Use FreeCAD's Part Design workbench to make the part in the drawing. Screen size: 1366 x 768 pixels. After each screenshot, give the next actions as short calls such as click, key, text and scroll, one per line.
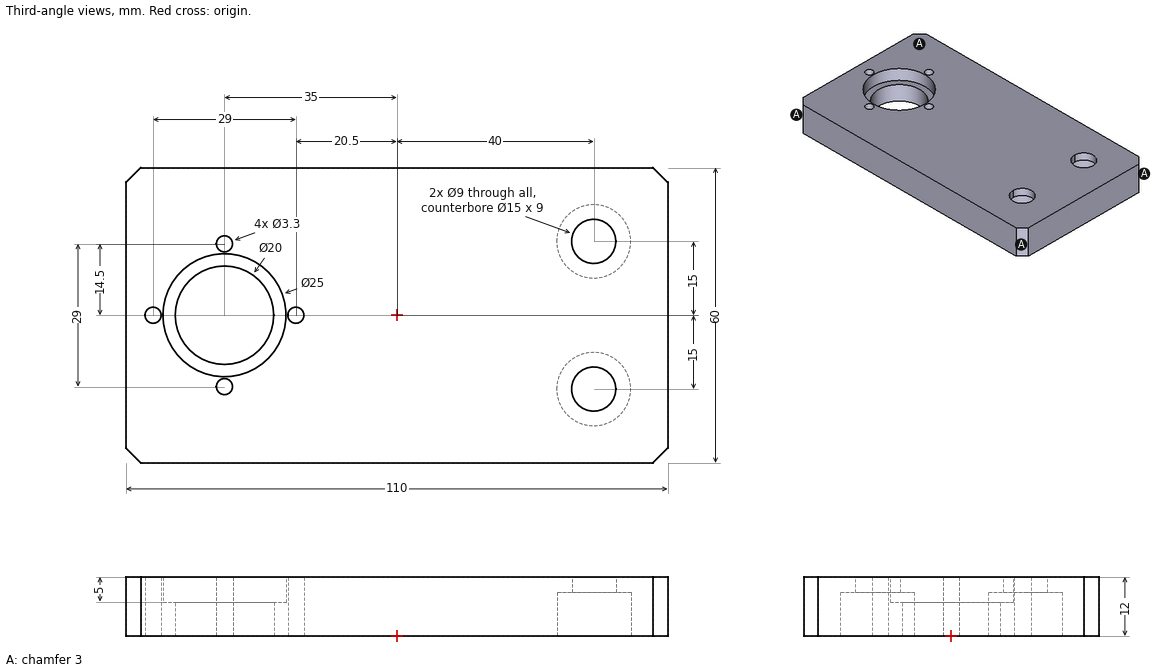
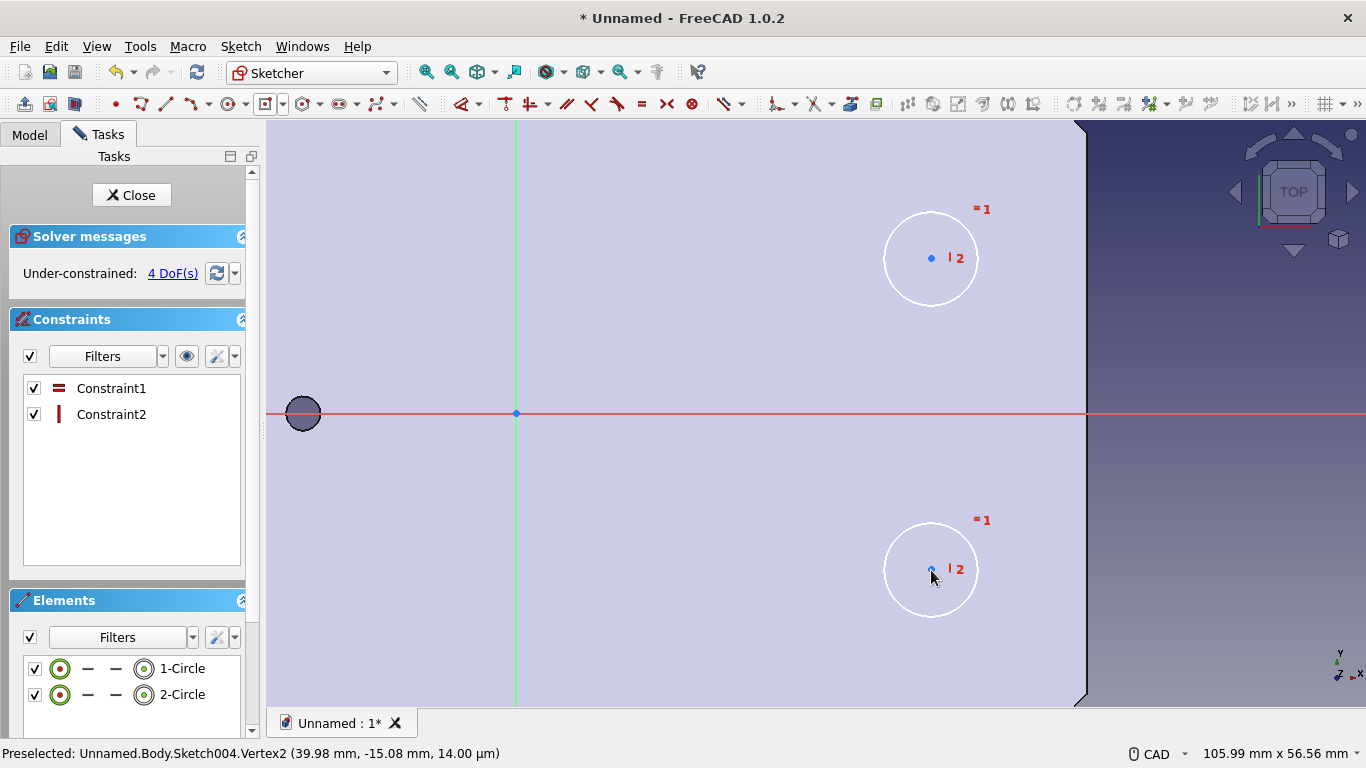
click(460, 104)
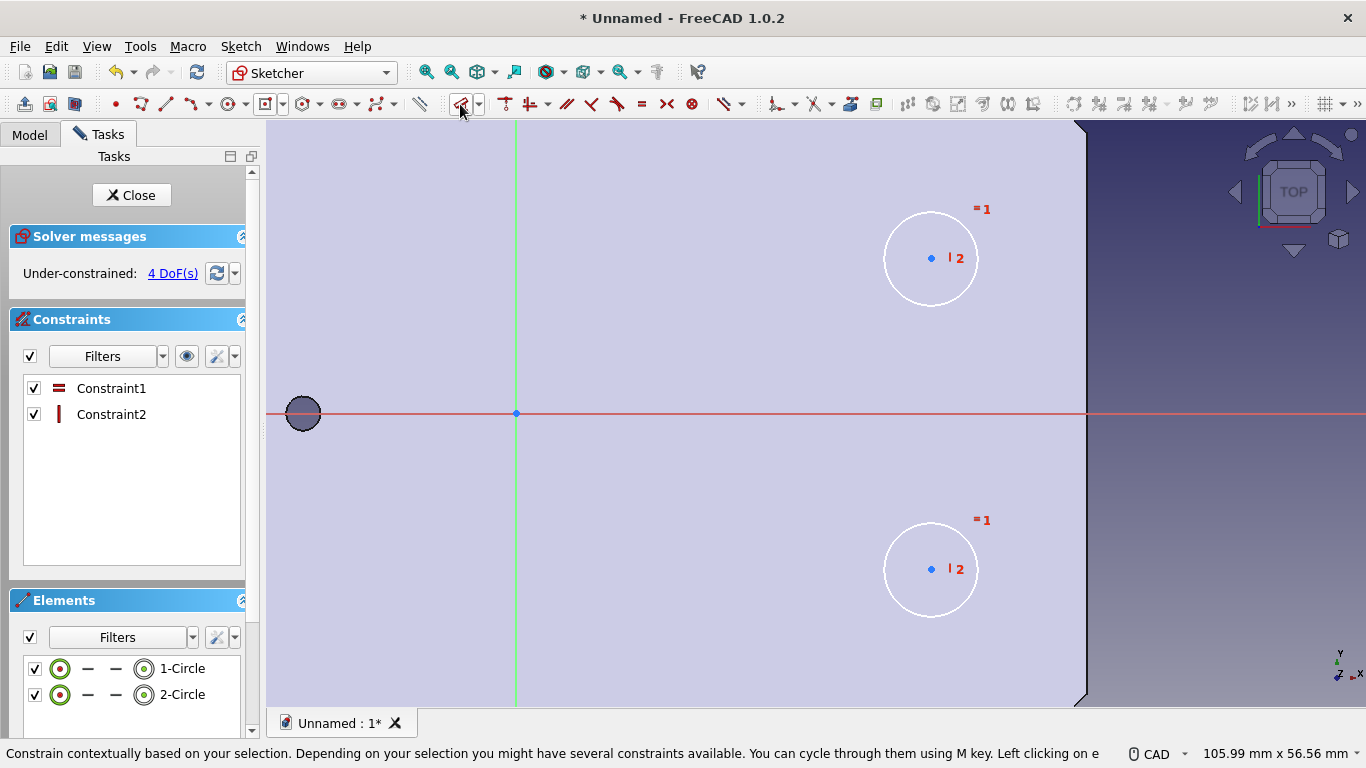
click(964, 226)
click(987, 203)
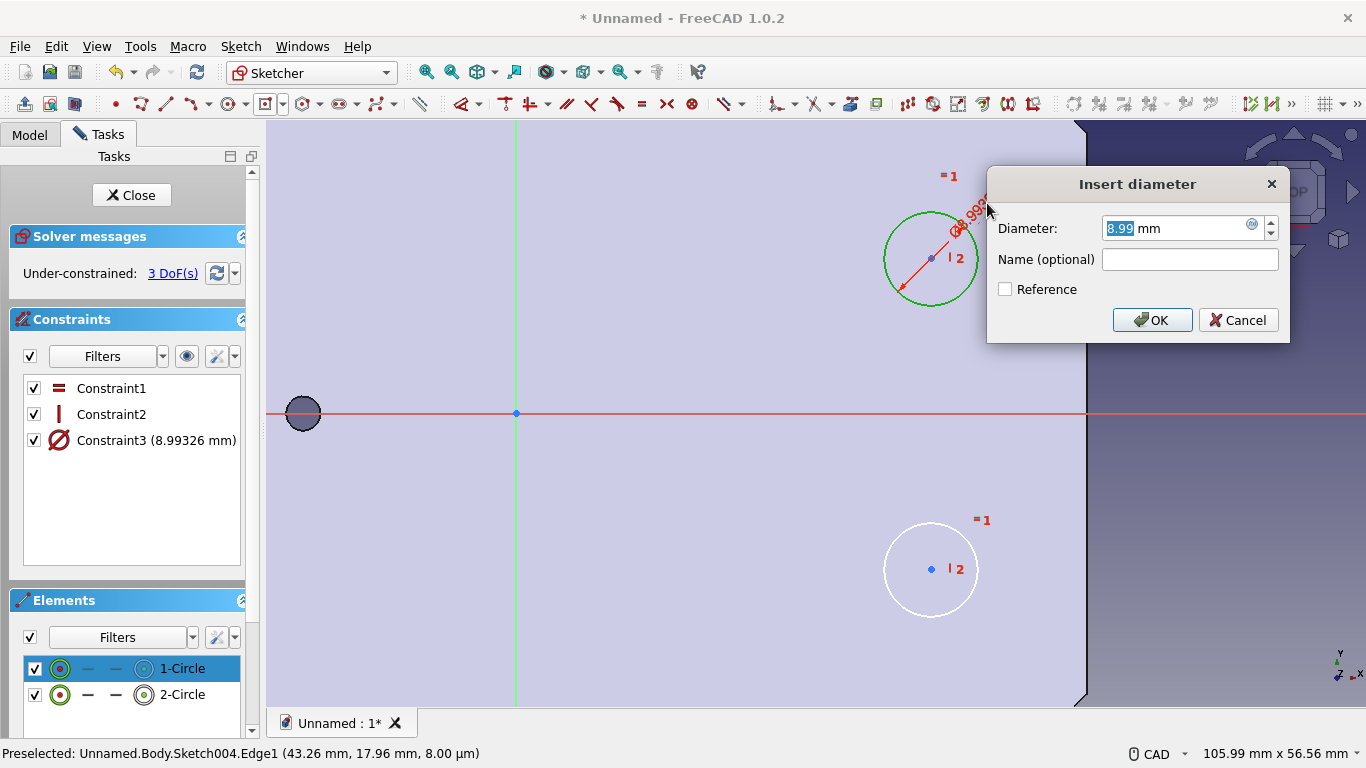
text(9)
key(Return)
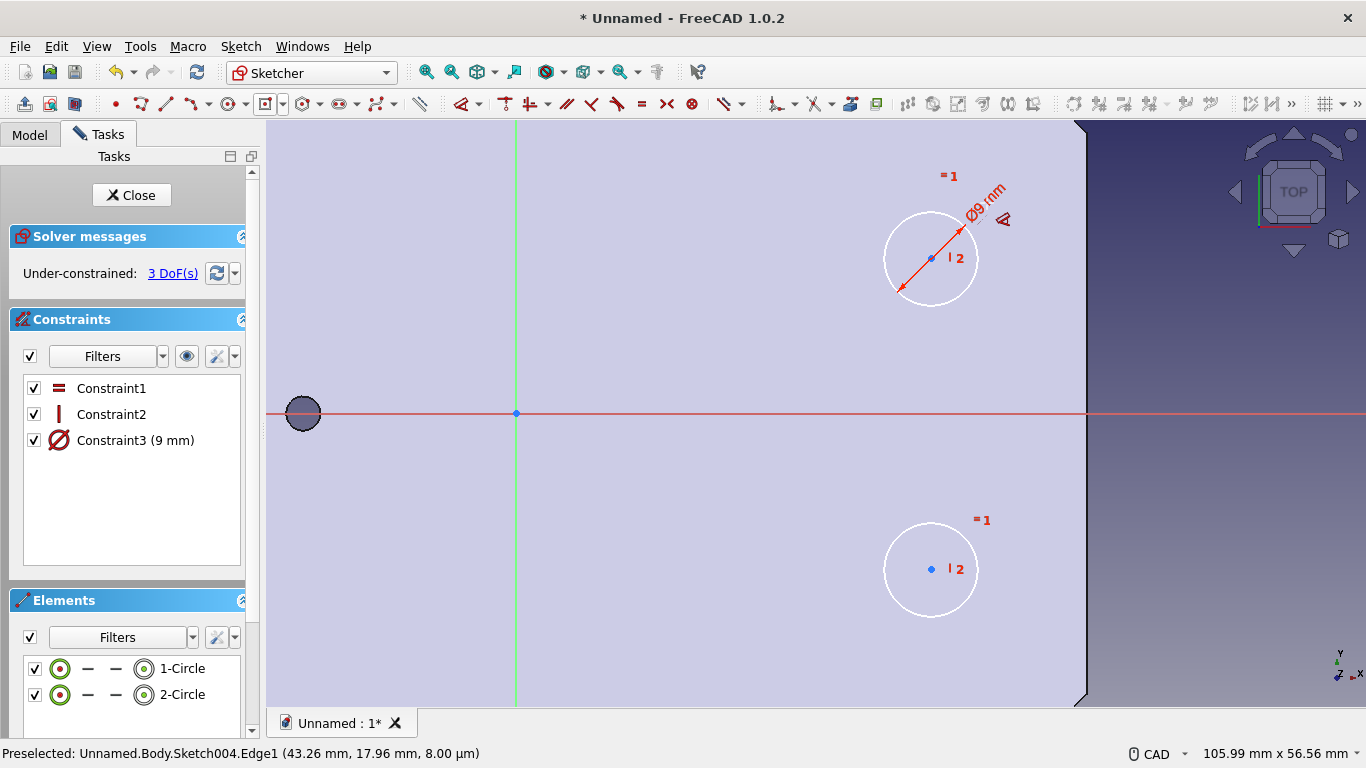
click(931, 259)
click(724, 225)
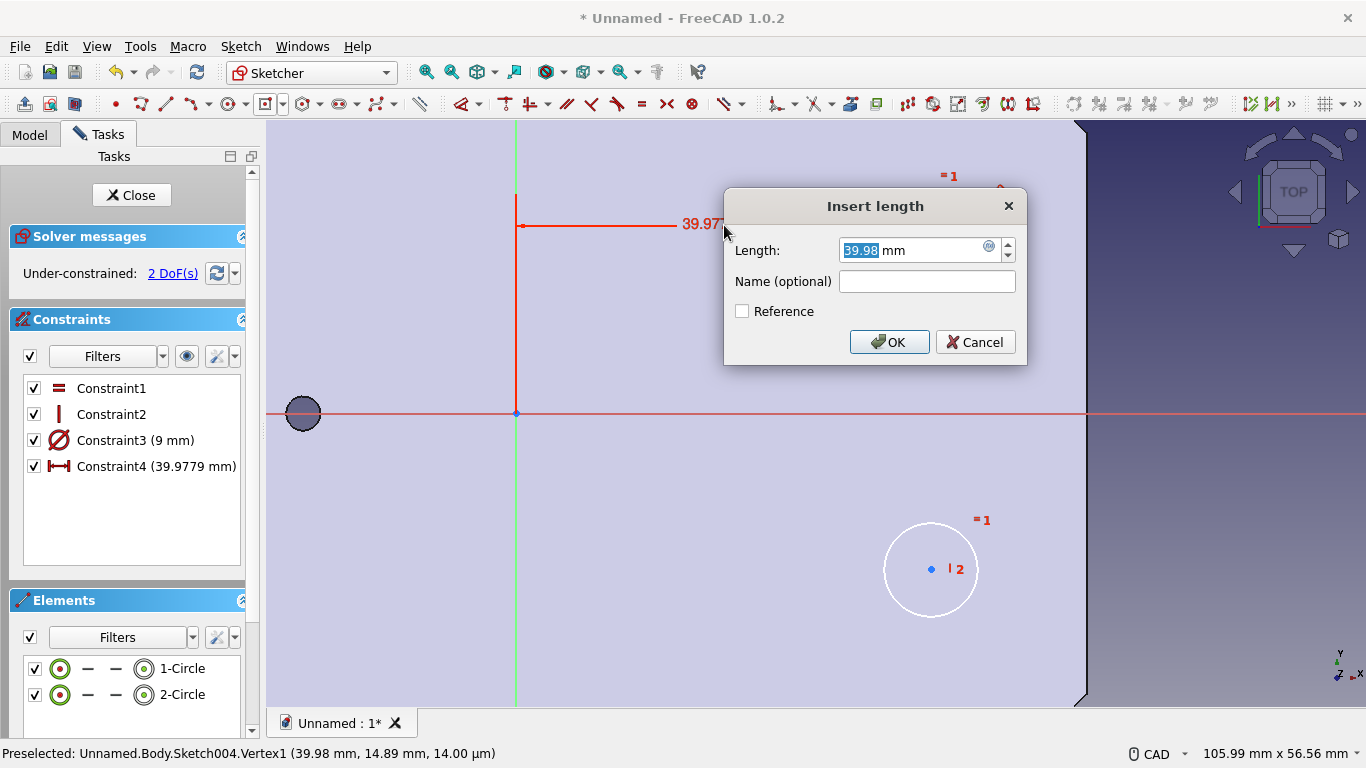
text(40)
key(Return)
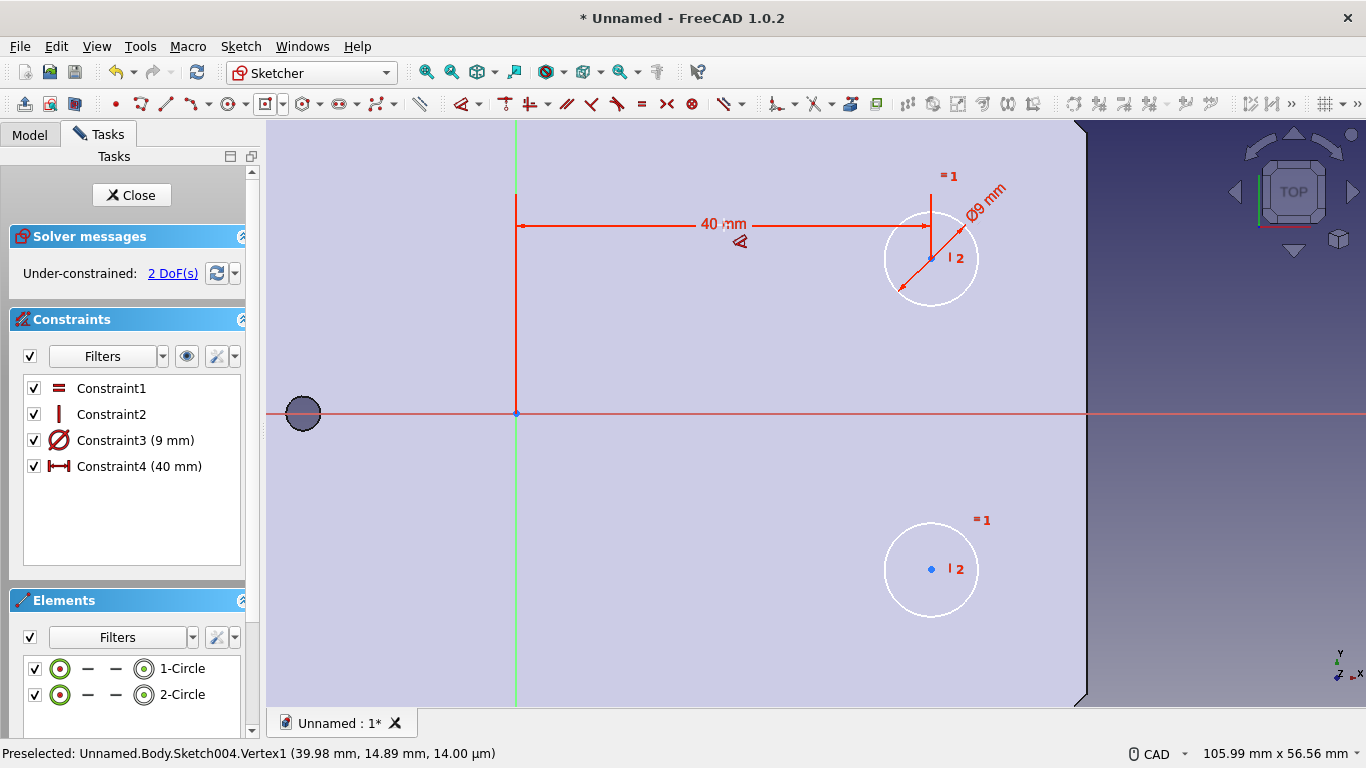
click(931, 259)
click(482, 336)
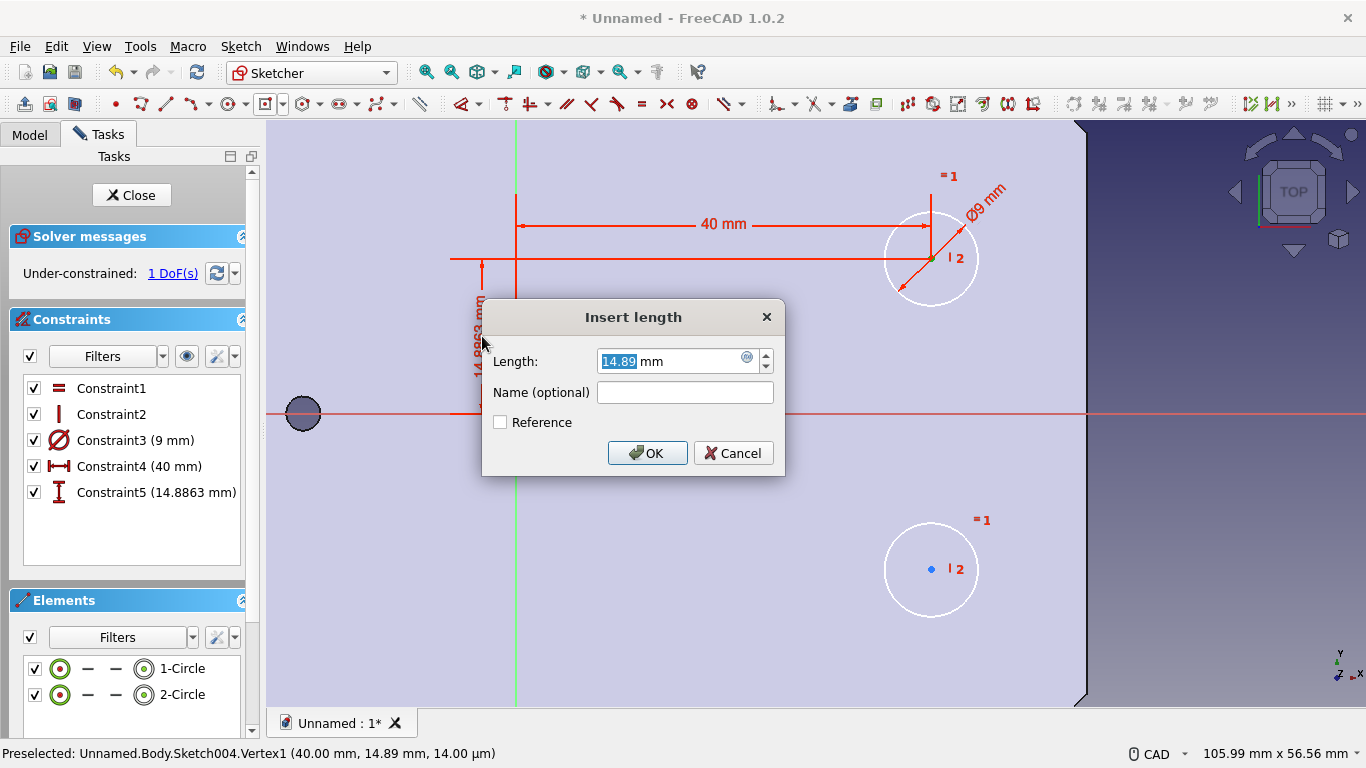
text(15)
key(Return)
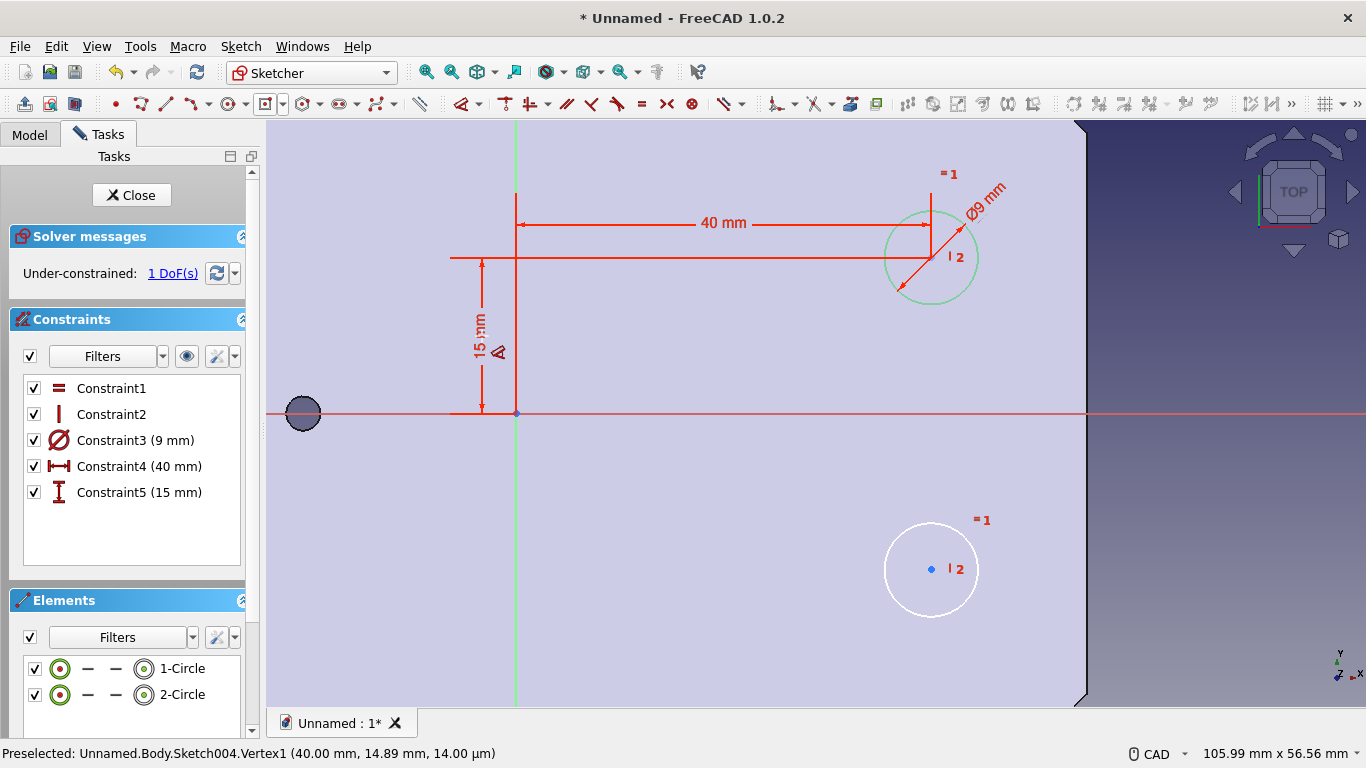
click(931, 570)
click(482, 492)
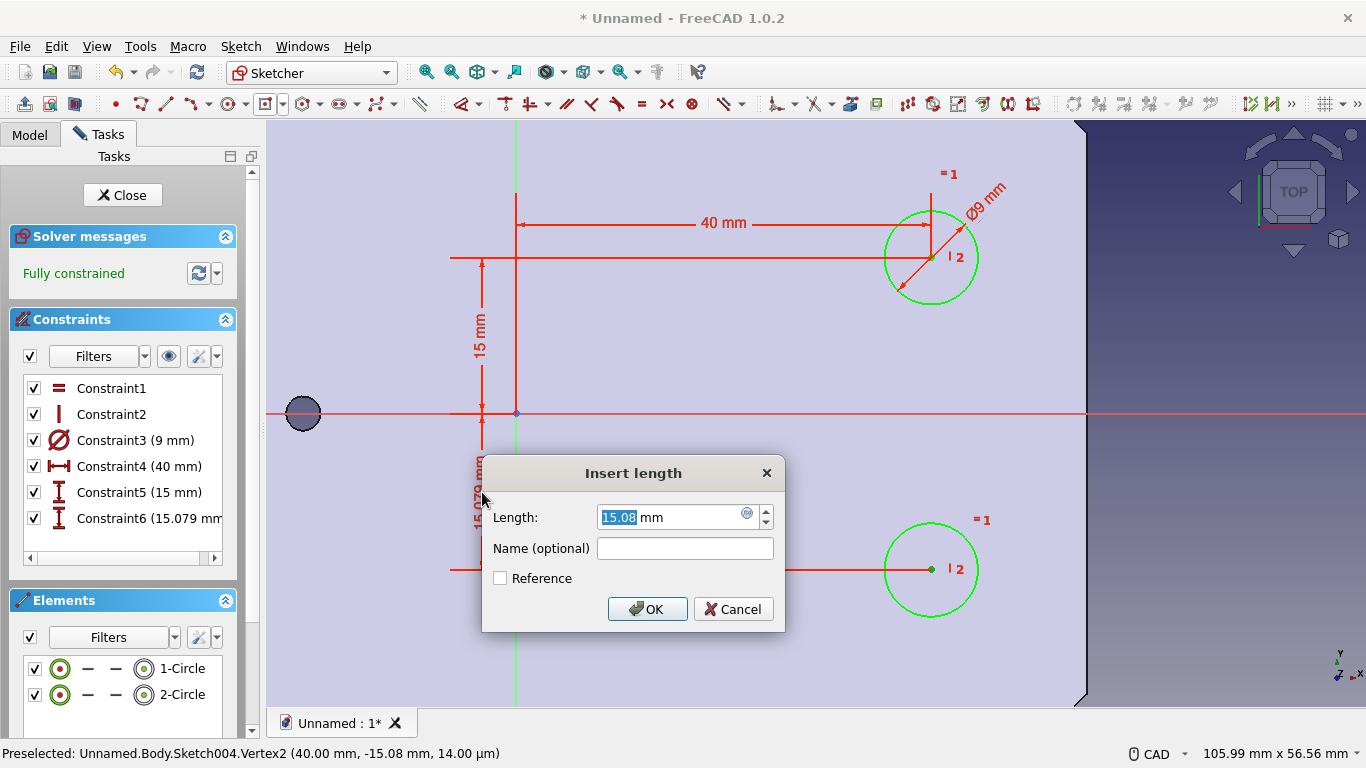
text(15)
key(Return)
key(Escape)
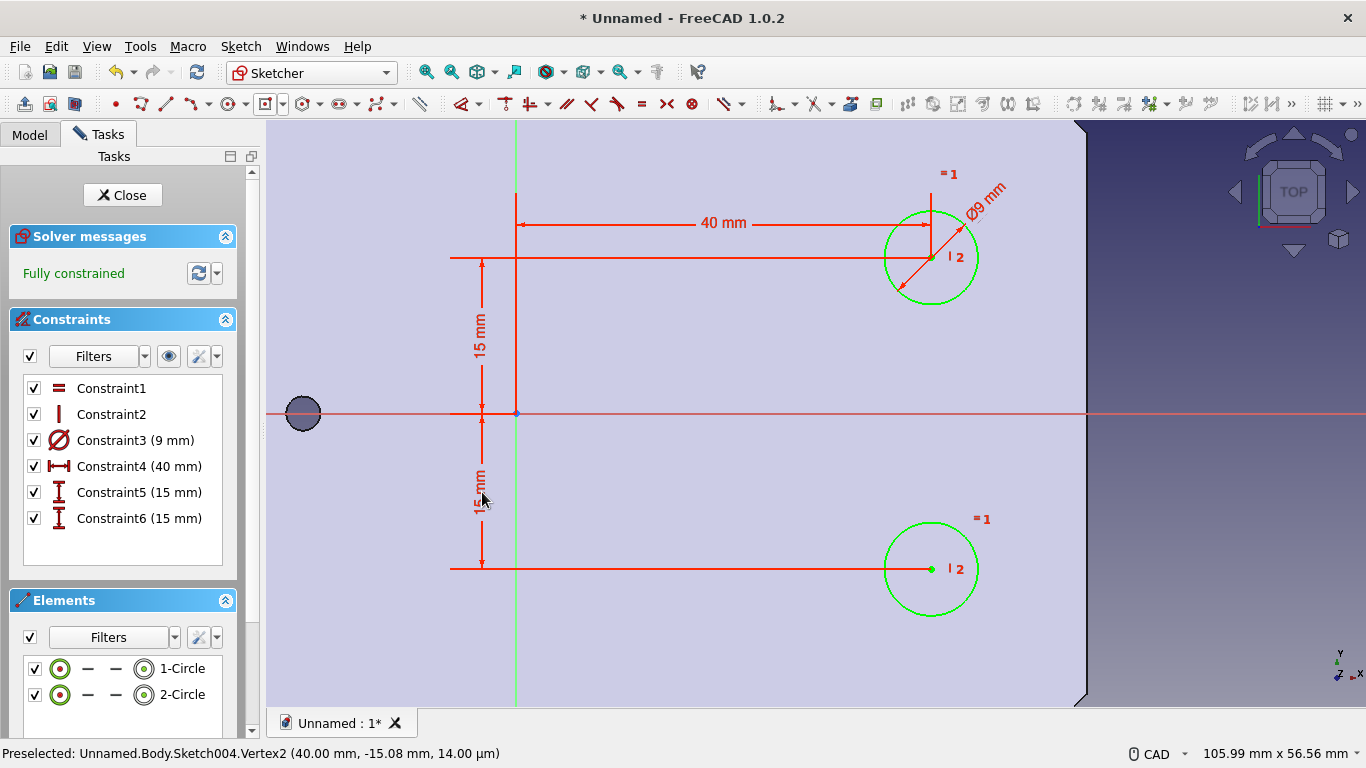
click(123, 195)